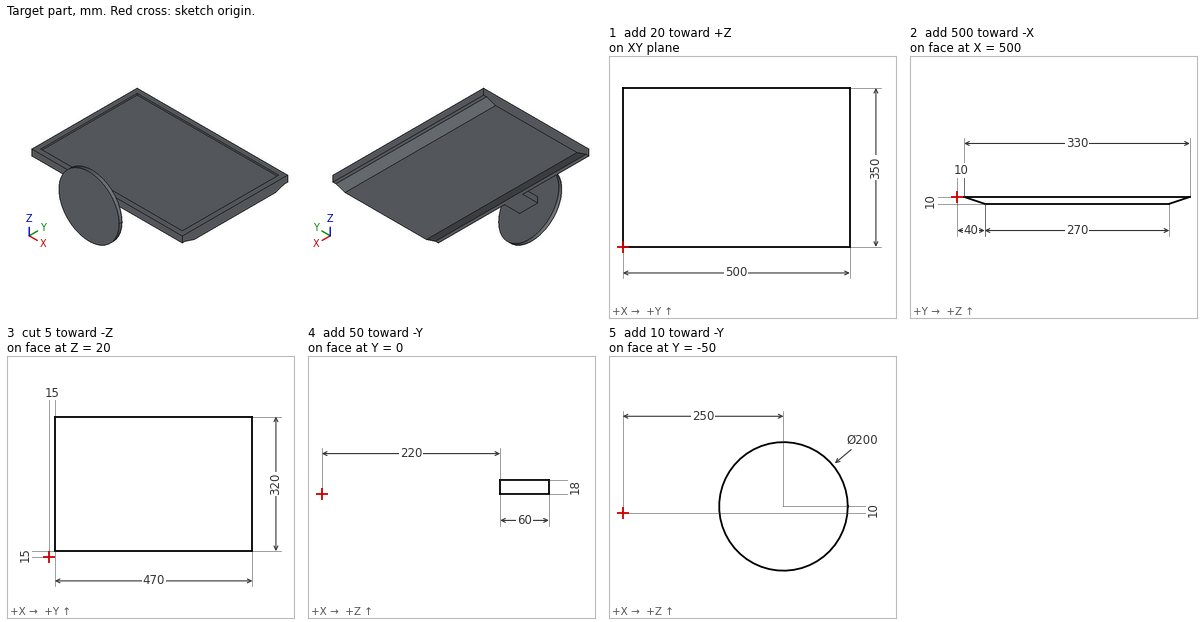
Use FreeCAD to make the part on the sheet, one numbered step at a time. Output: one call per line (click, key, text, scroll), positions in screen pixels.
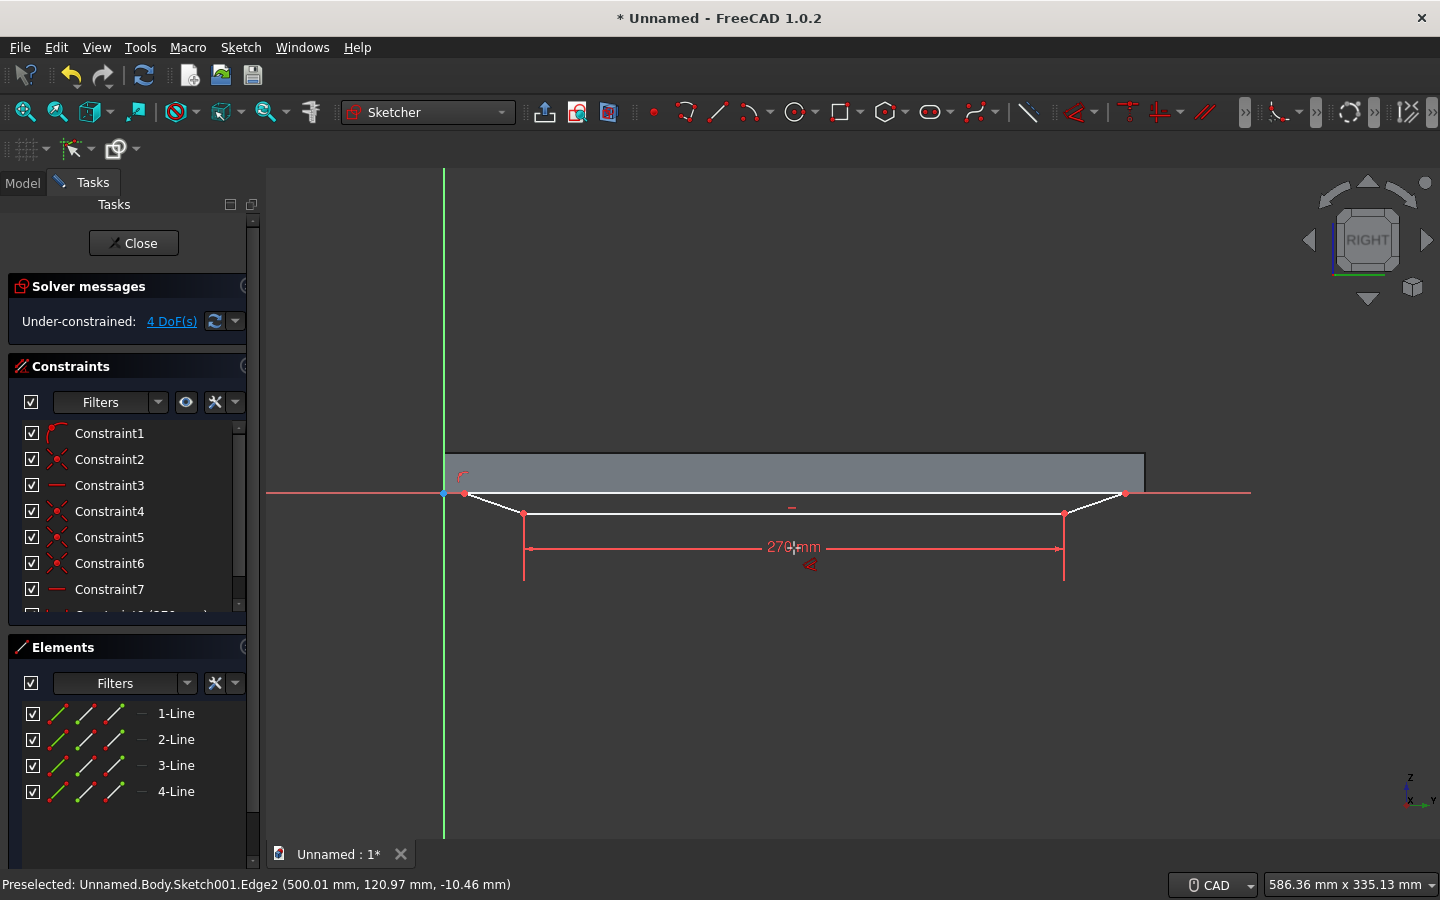
click(927, 493)
click(794, 459)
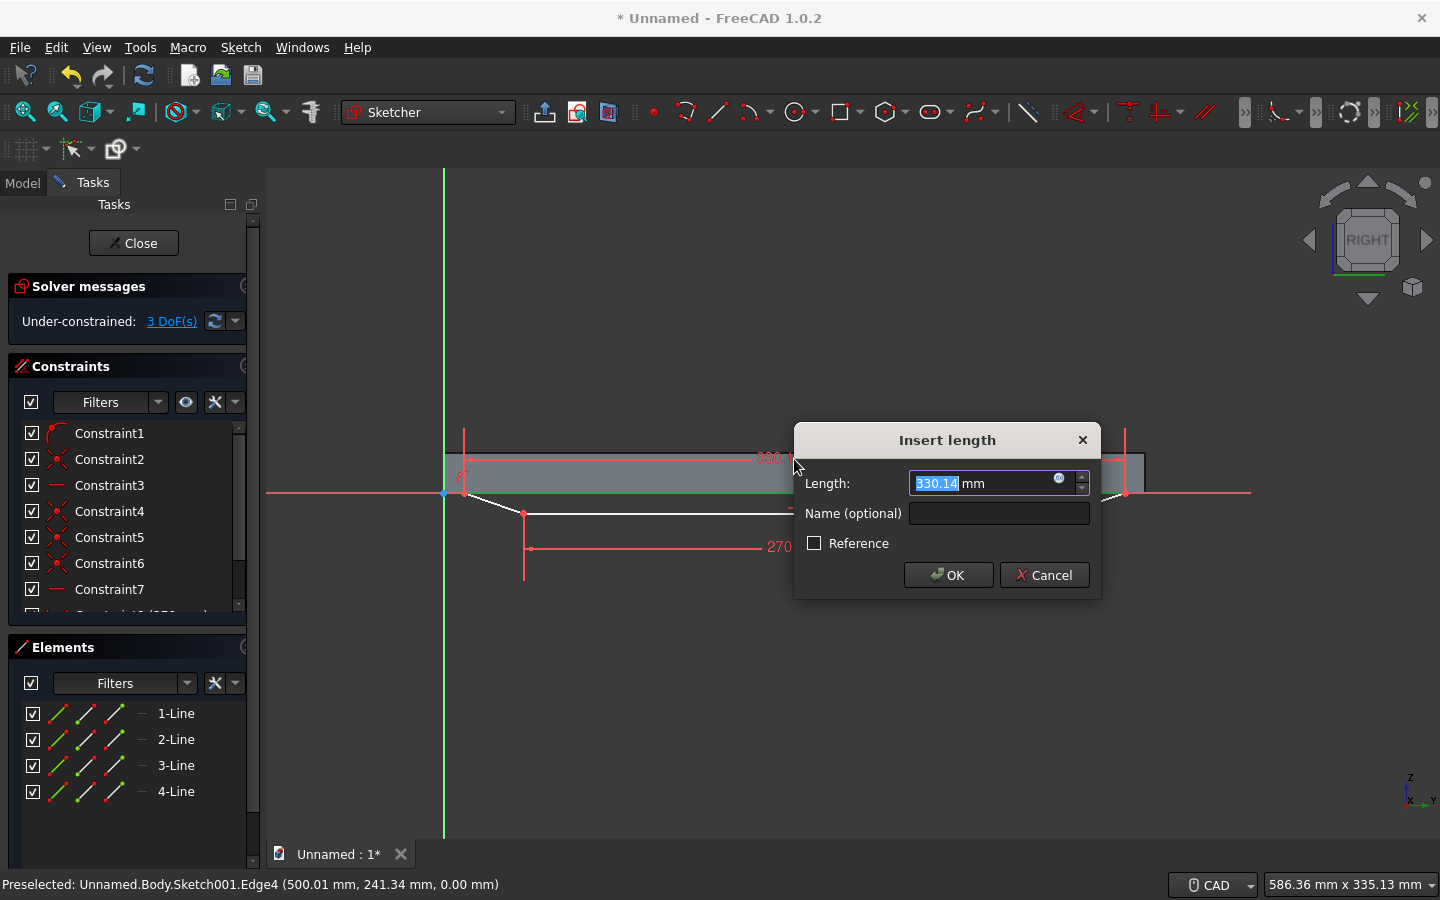
text(330)
key(Return)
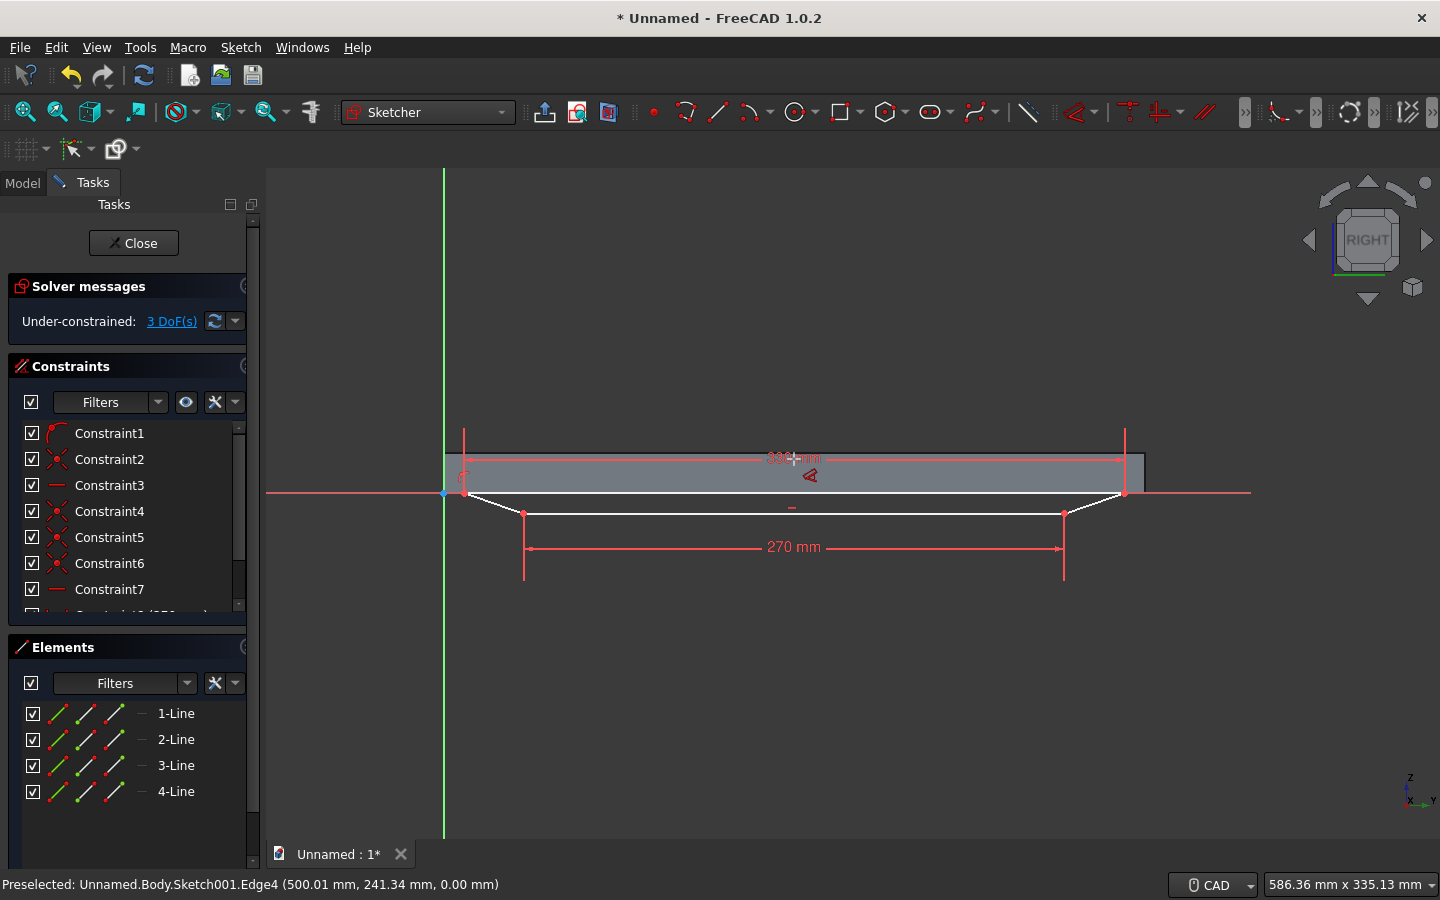
scroll(464, 493, up, 4)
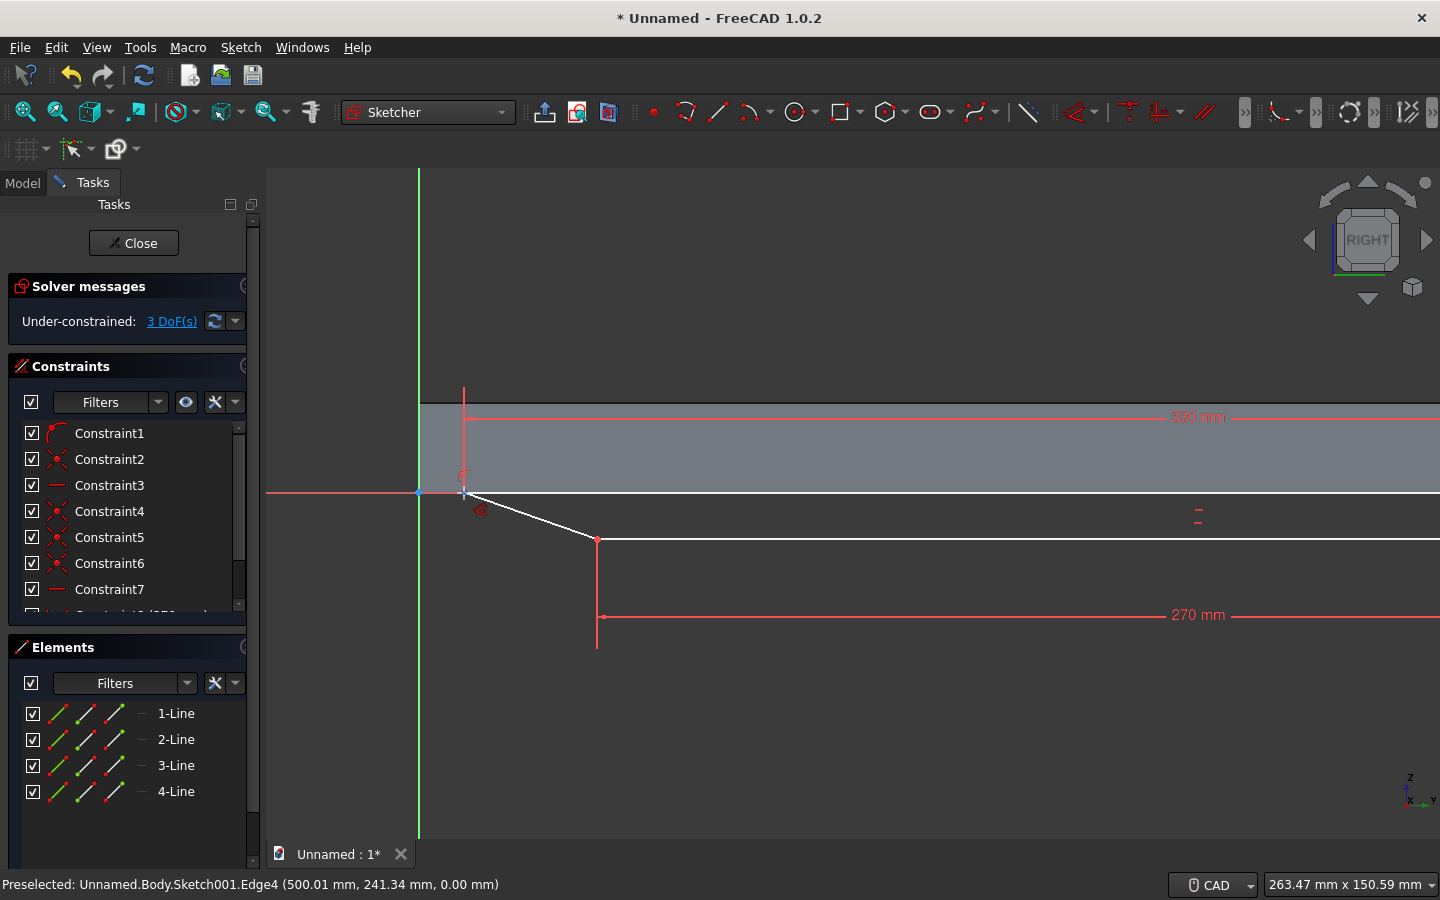
click(464, 493)
click(441, 459)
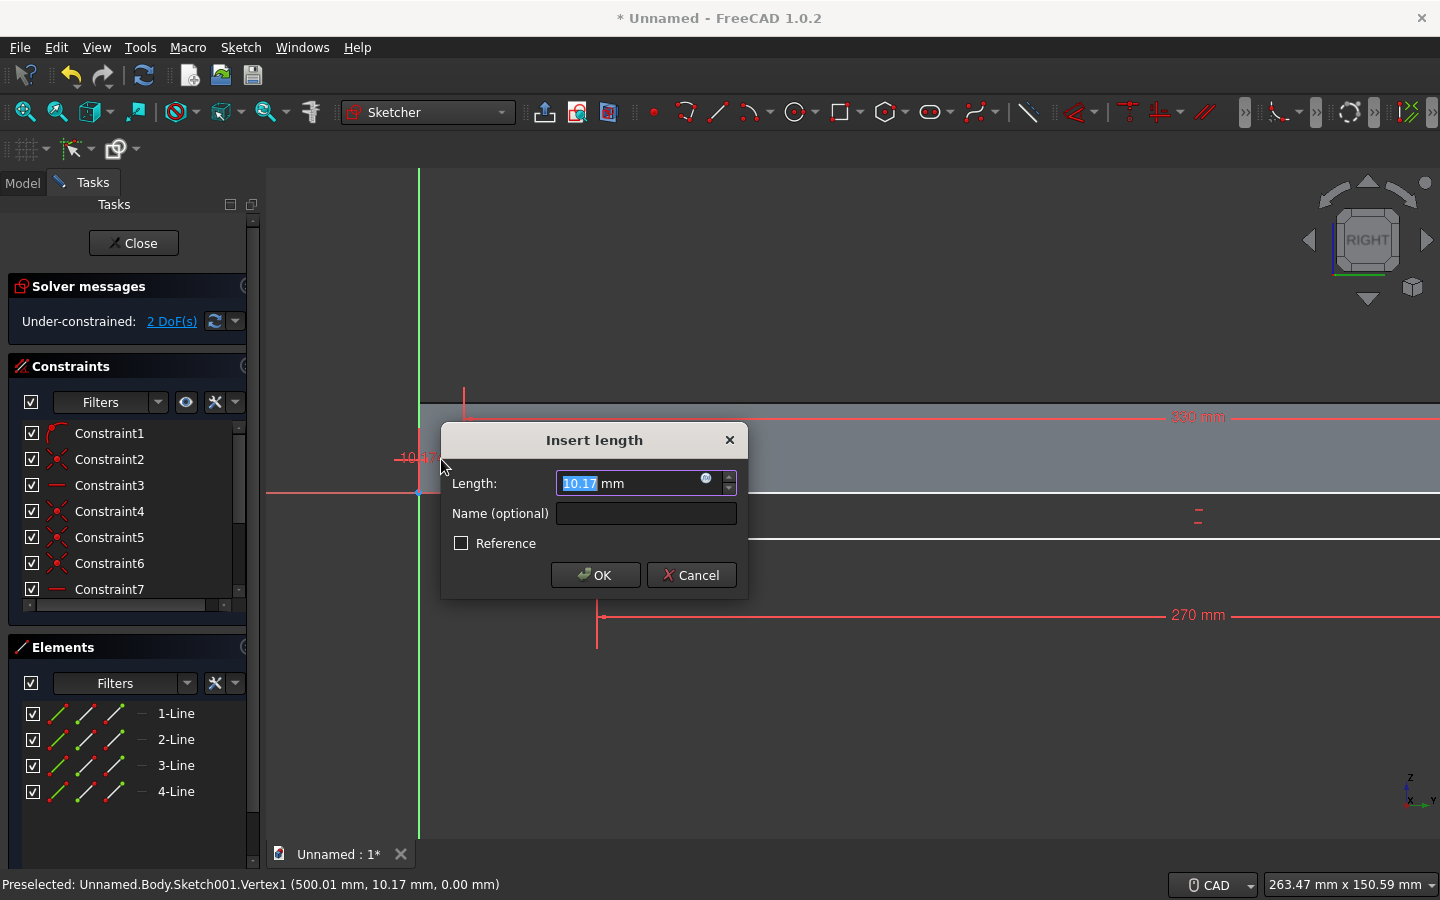
text(10)
key(Return)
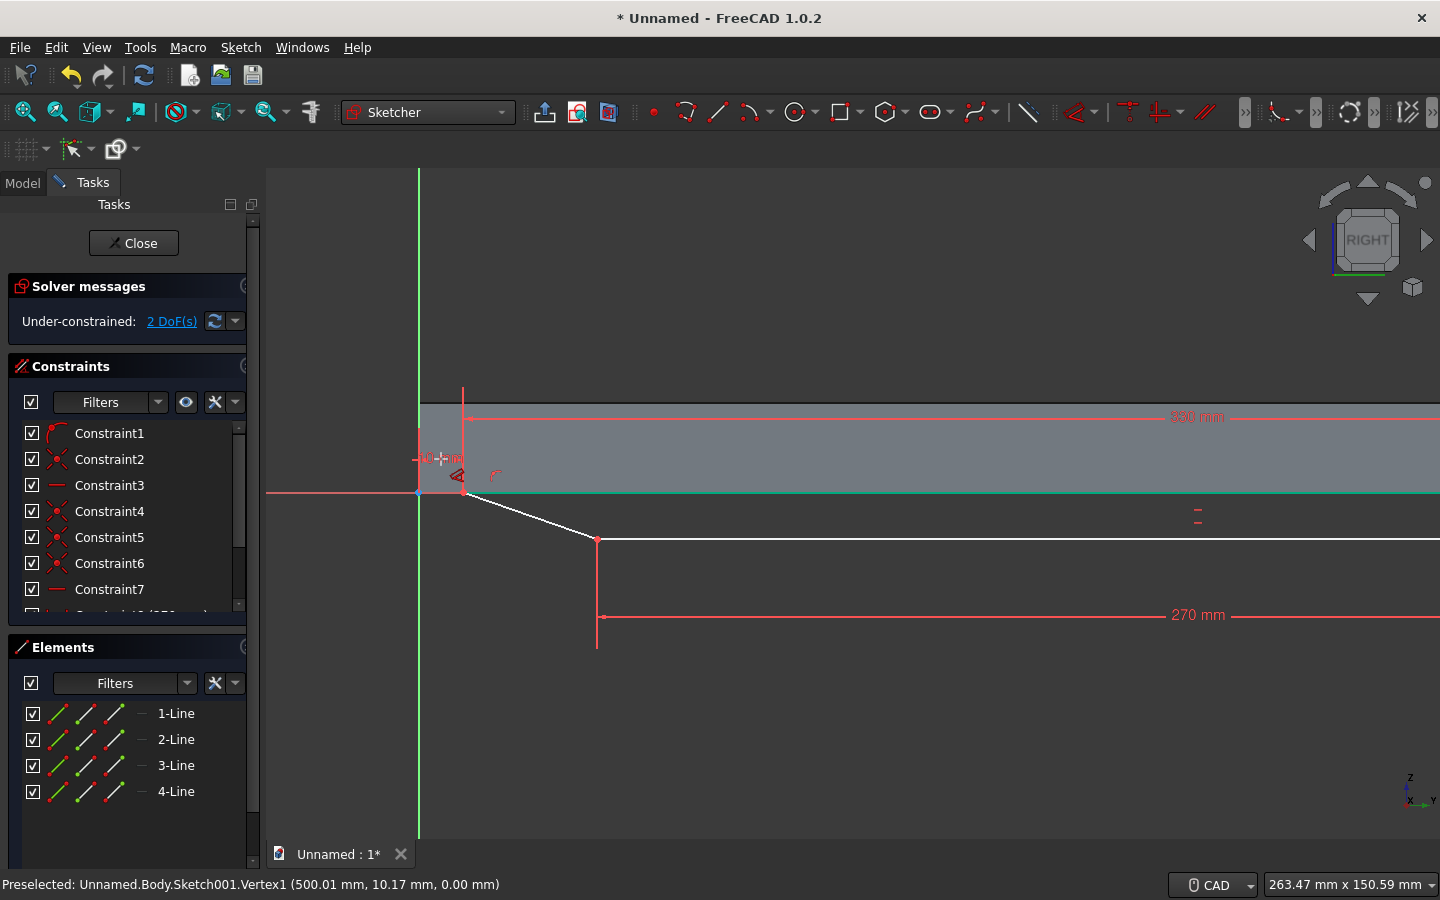
click(597, 539)
click(508, 573)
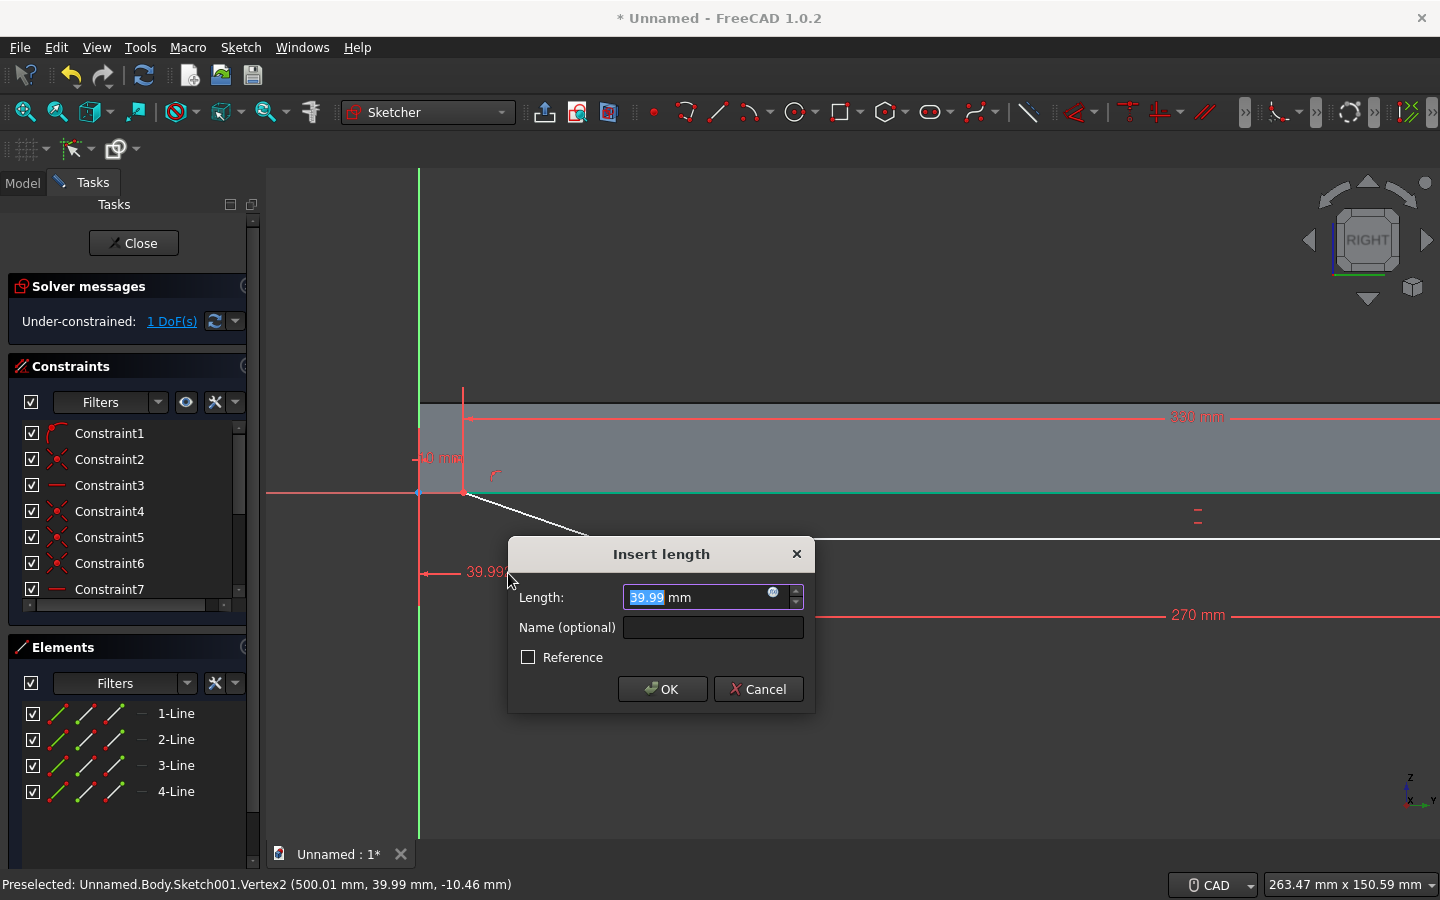
text(40)
key(Return)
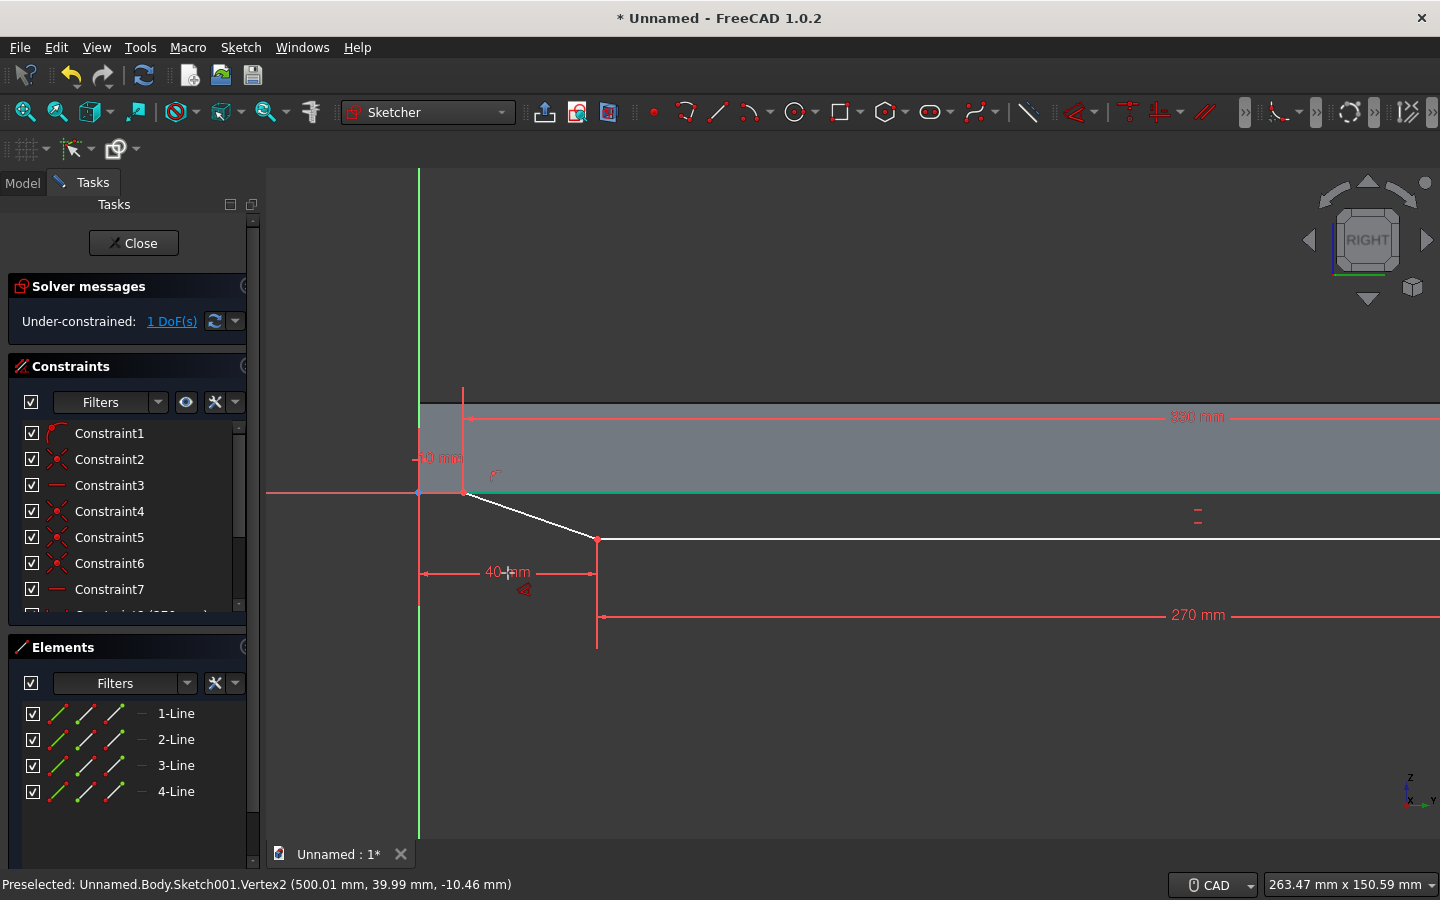
click(597, 539)
click(385, 516)